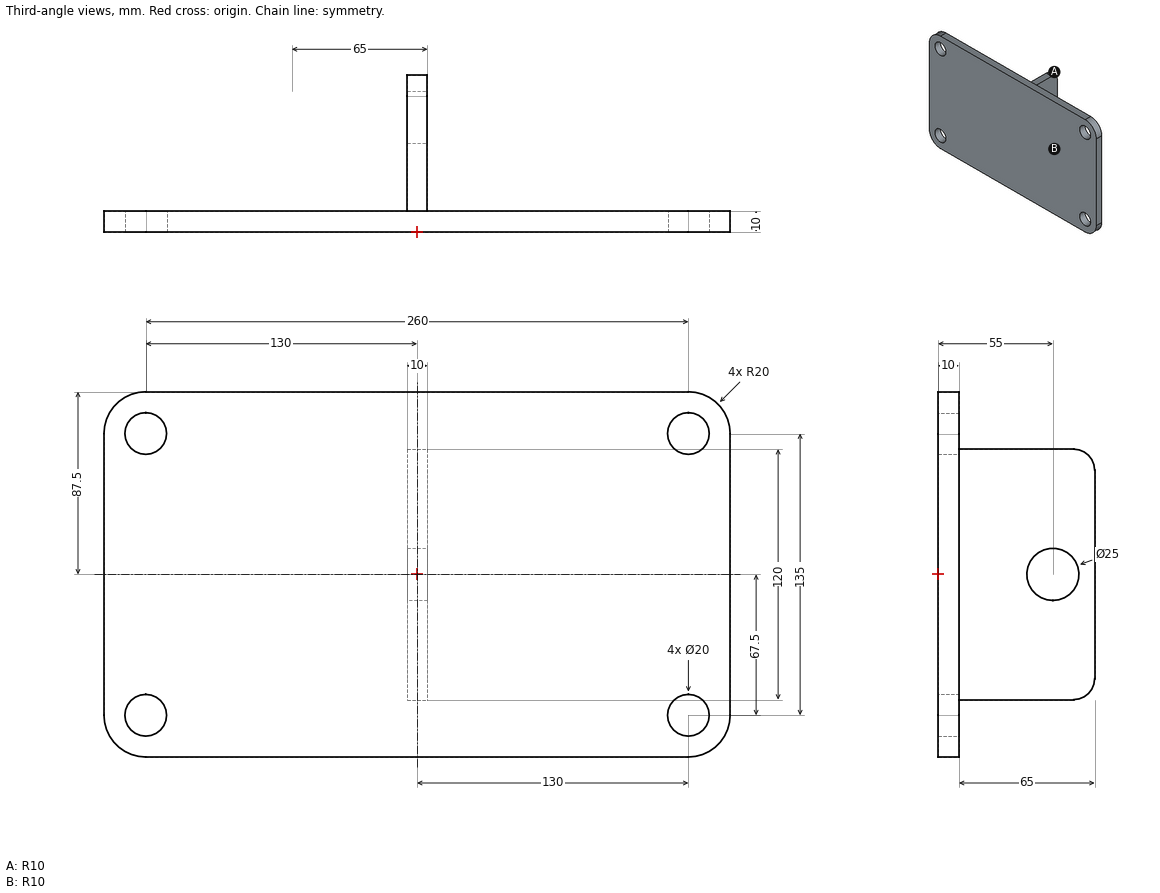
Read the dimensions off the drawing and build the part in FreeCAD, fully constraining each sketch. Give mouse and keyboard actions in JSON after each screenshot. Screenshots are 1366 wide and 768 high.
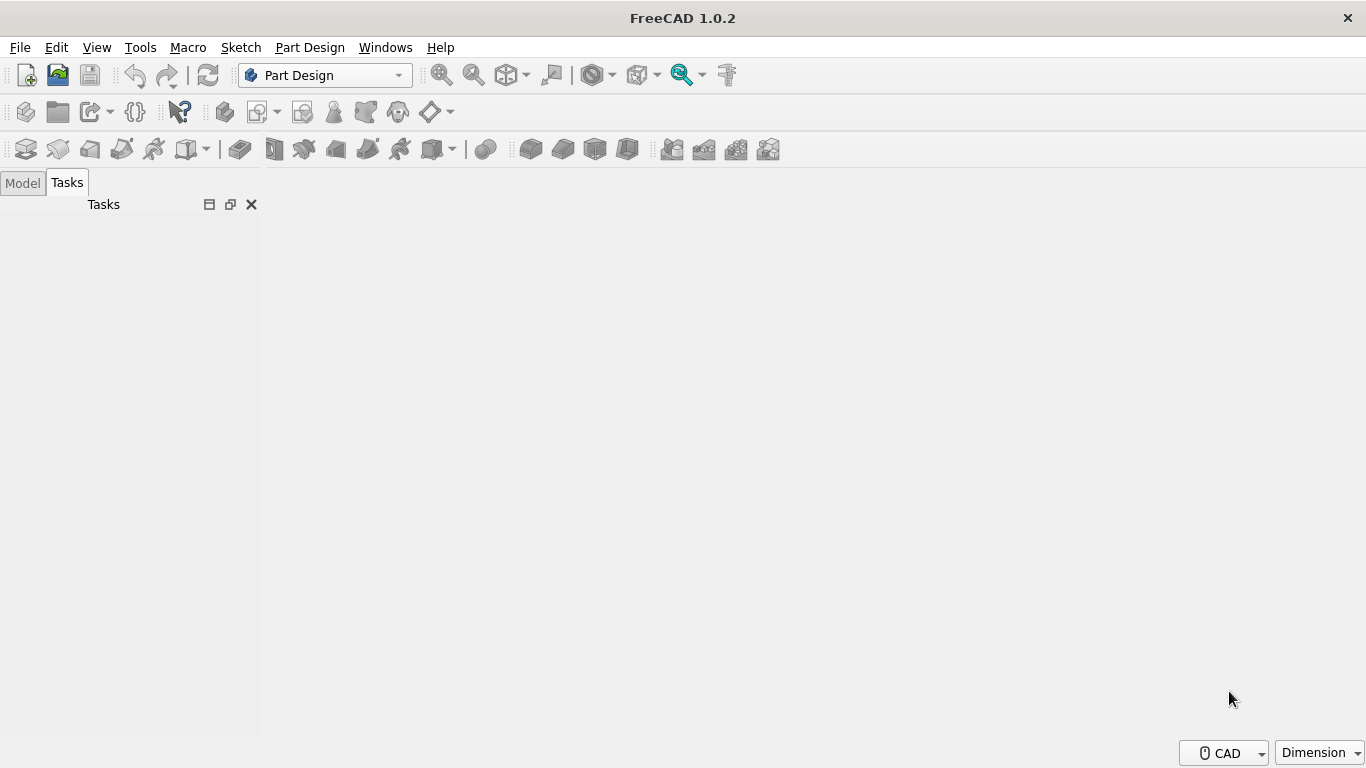
{"action": "left_click", "coordinate": [576, 112]}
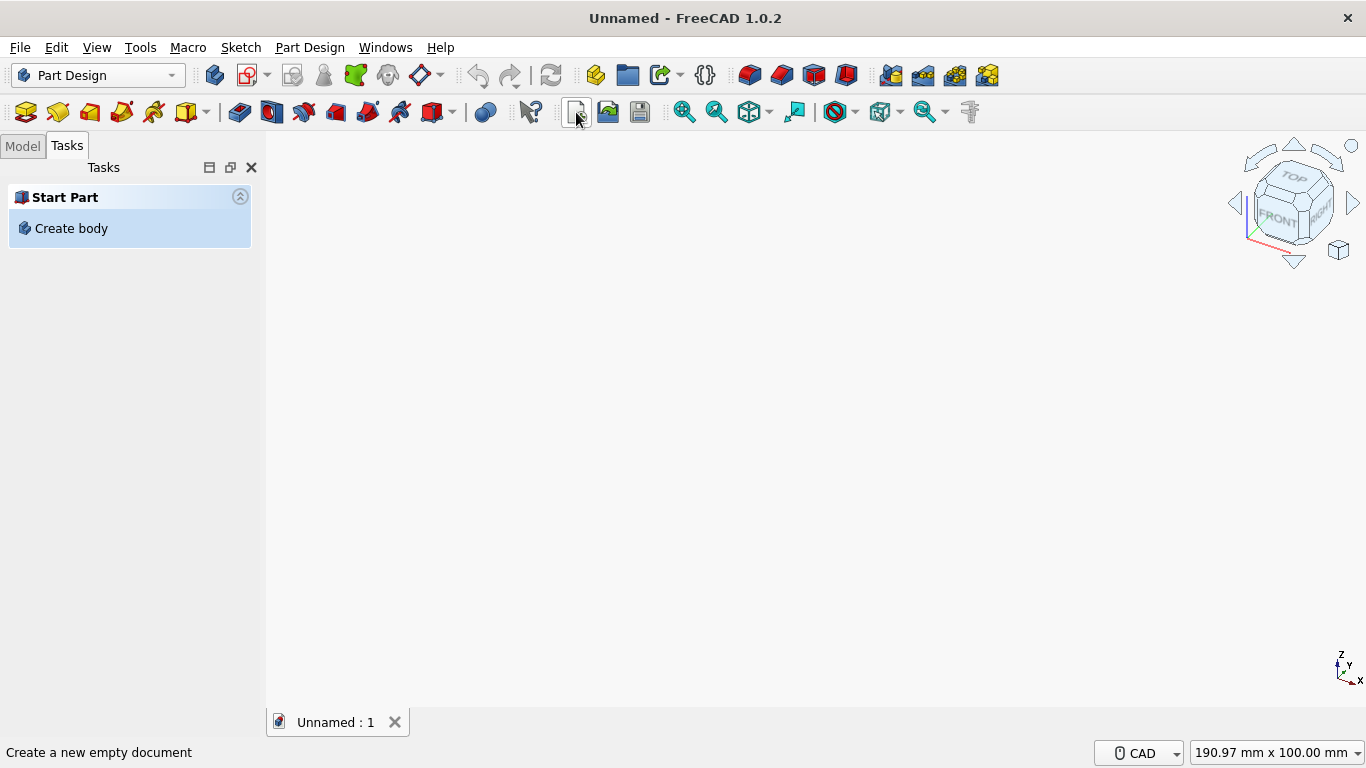
{"action": "left_click", "coordinate": [248, 76]}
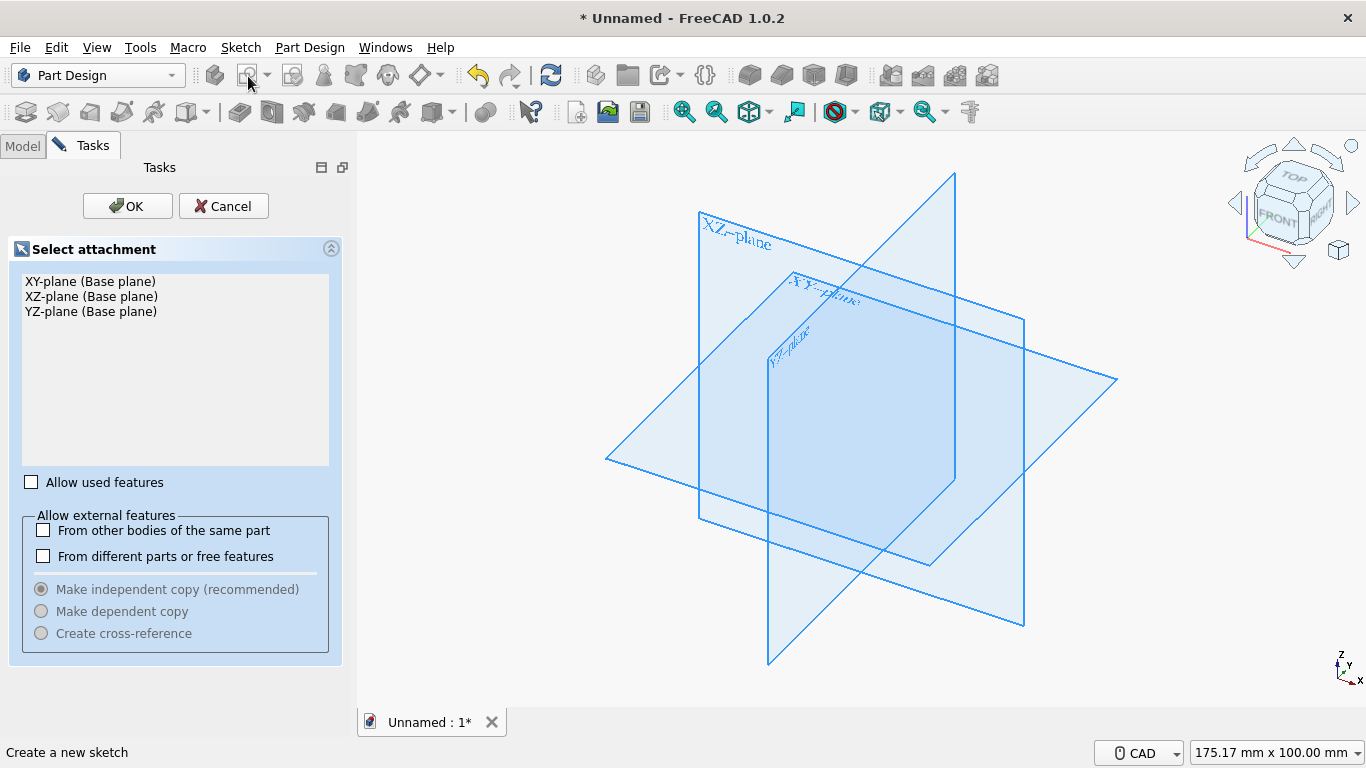
{"action": "left_click", "coordinate": [82, 296]}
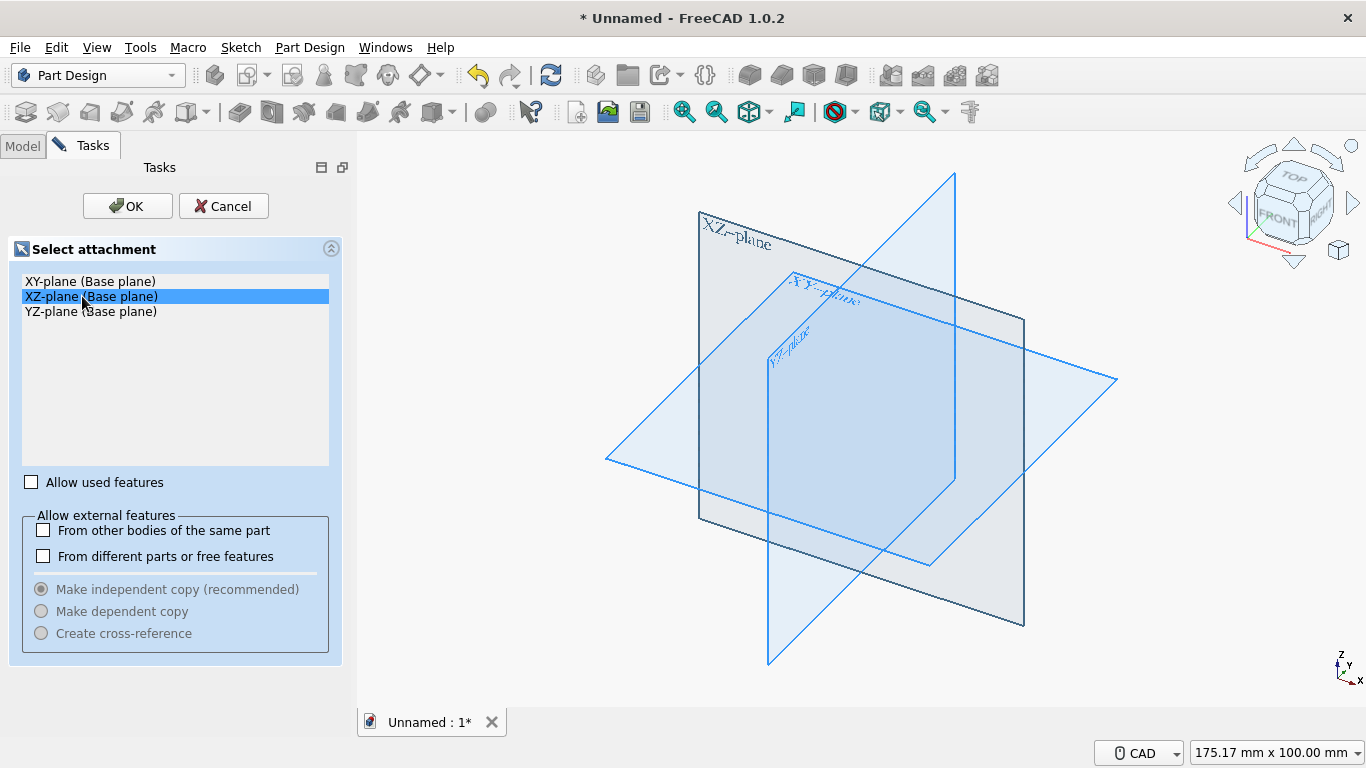
{"action": "left_click", "coordinate": [128, 206]}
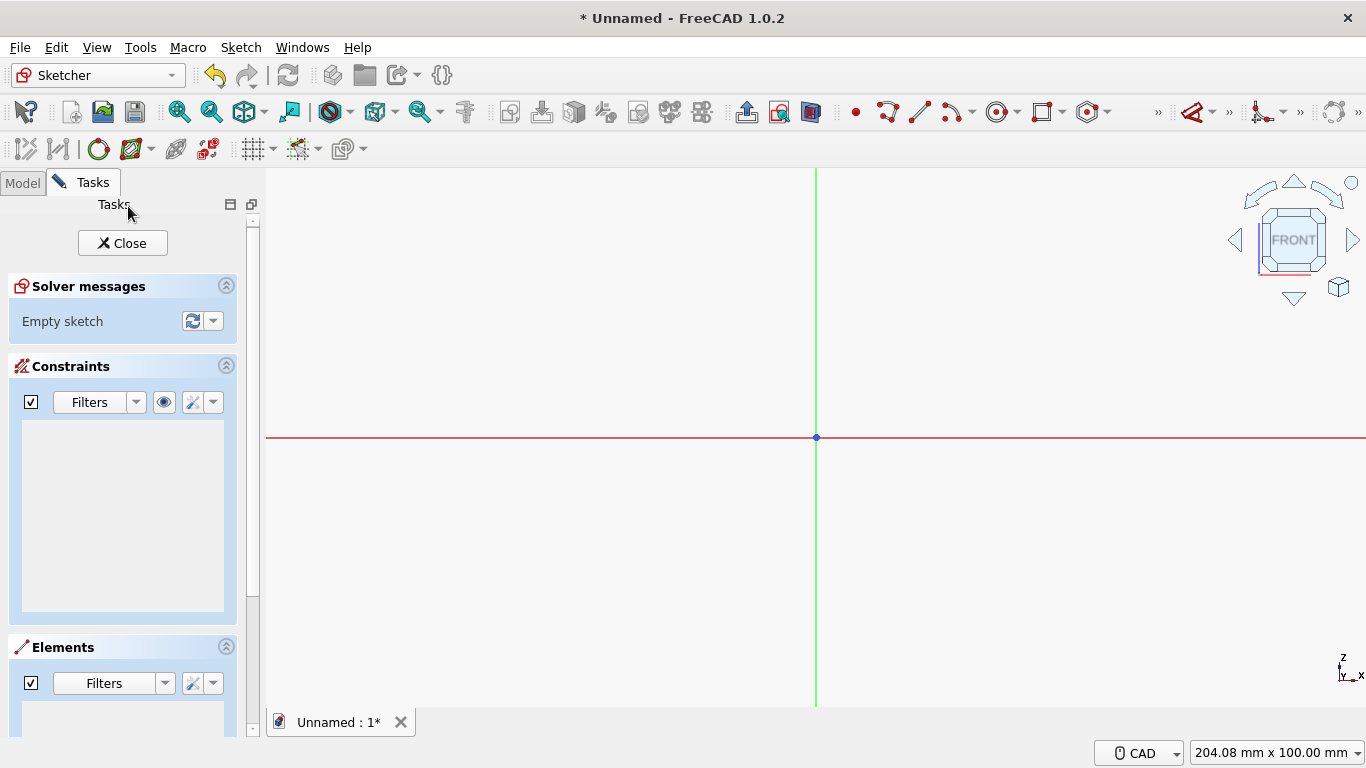
{"action": "scroll", "coordinate": [708, 438], "scroll_direction": "down", "scroll_amount": 5}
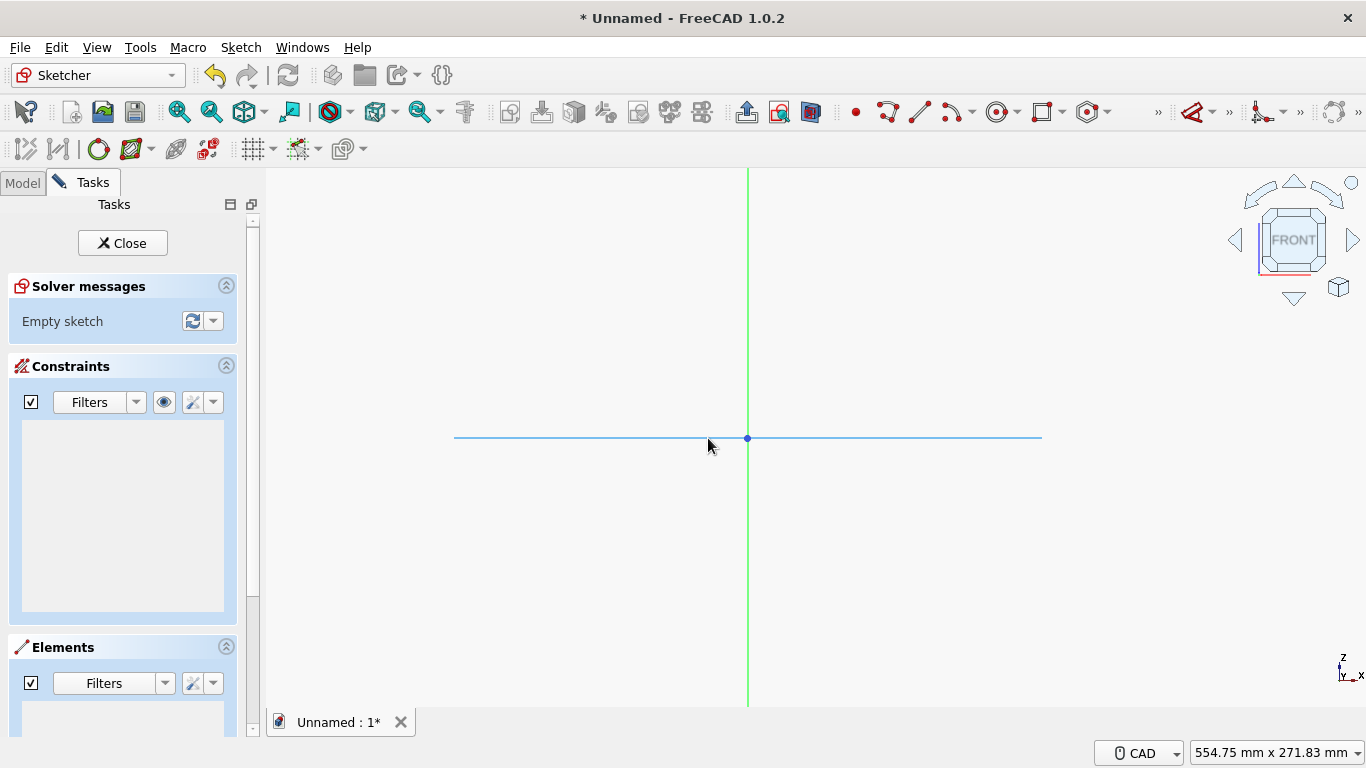
{"action": "left_click", "coordinate": [920, 112]}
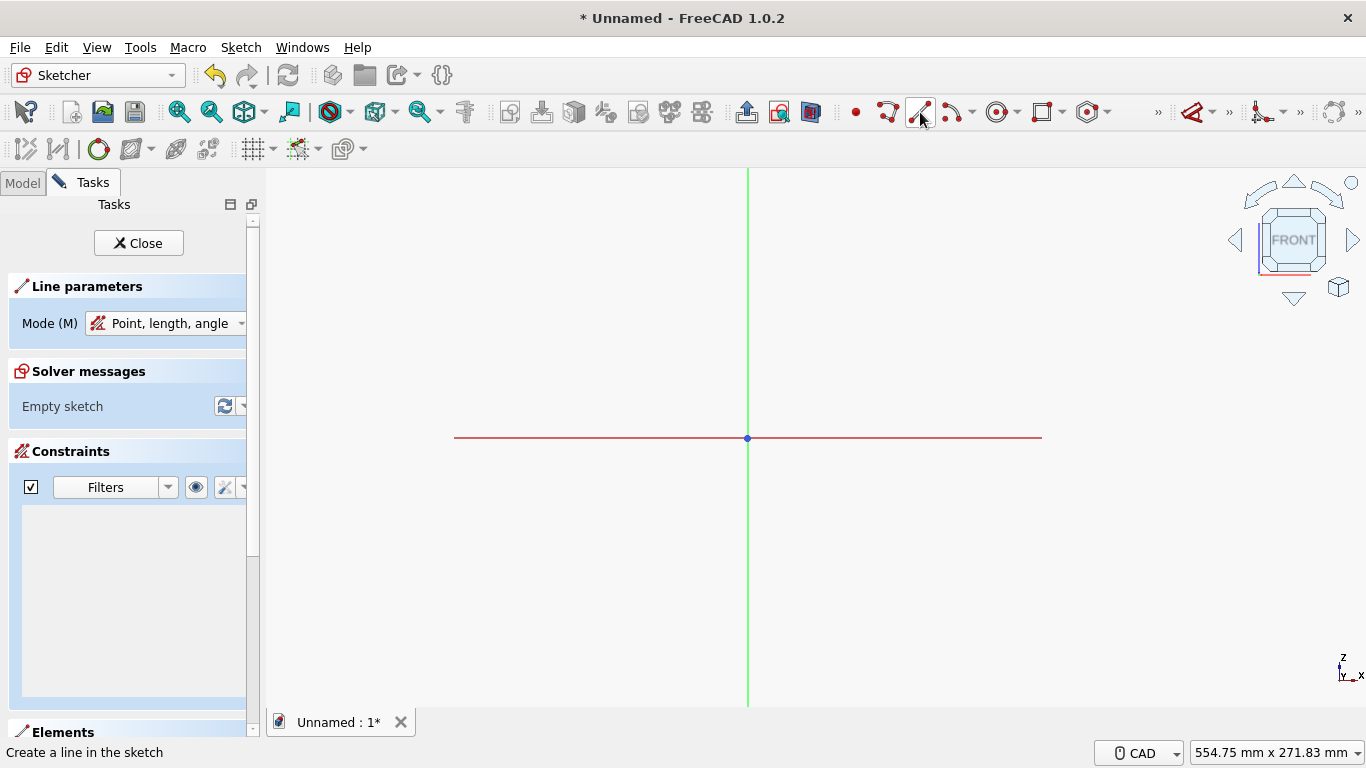
{"action": "left_click", "coordinate": [490, 265]}
{"action": "left_click", "coordinate": [1006, 265]}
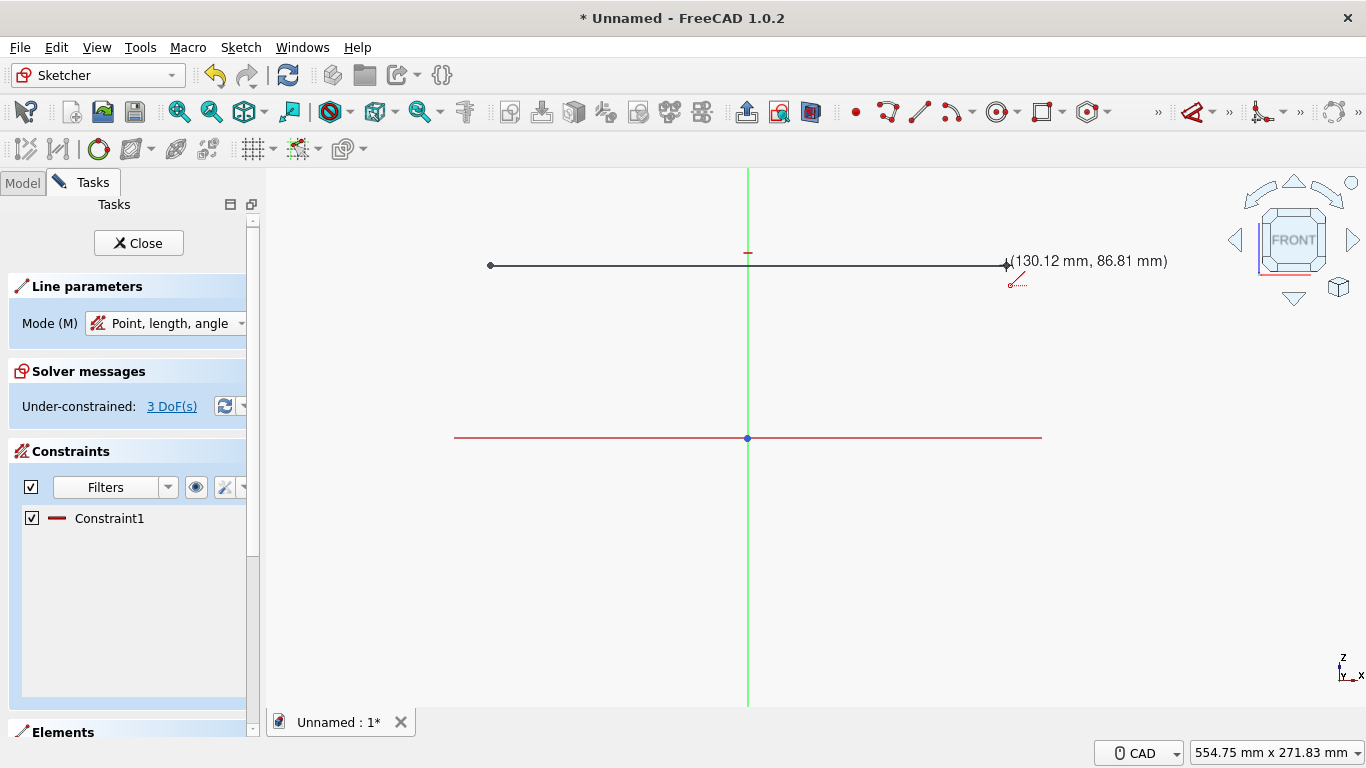
{"action": "left_click", "coordinate": [1045, 304]}
{"action": "left_click", "coordinate": [1045, 572]}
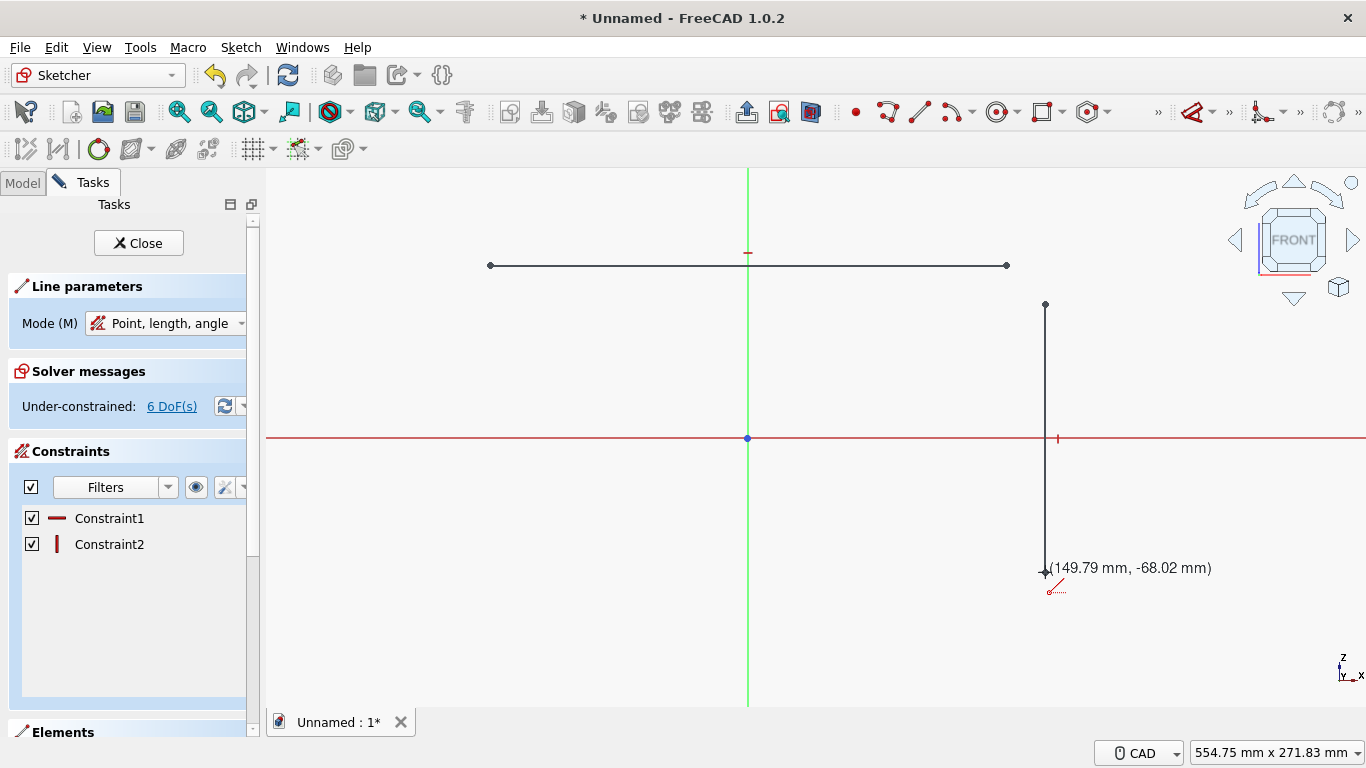
{"action": "left_click", "coordinate": [1006, 612]}
{"action": "left_click", "coordinate": [490, 612]}